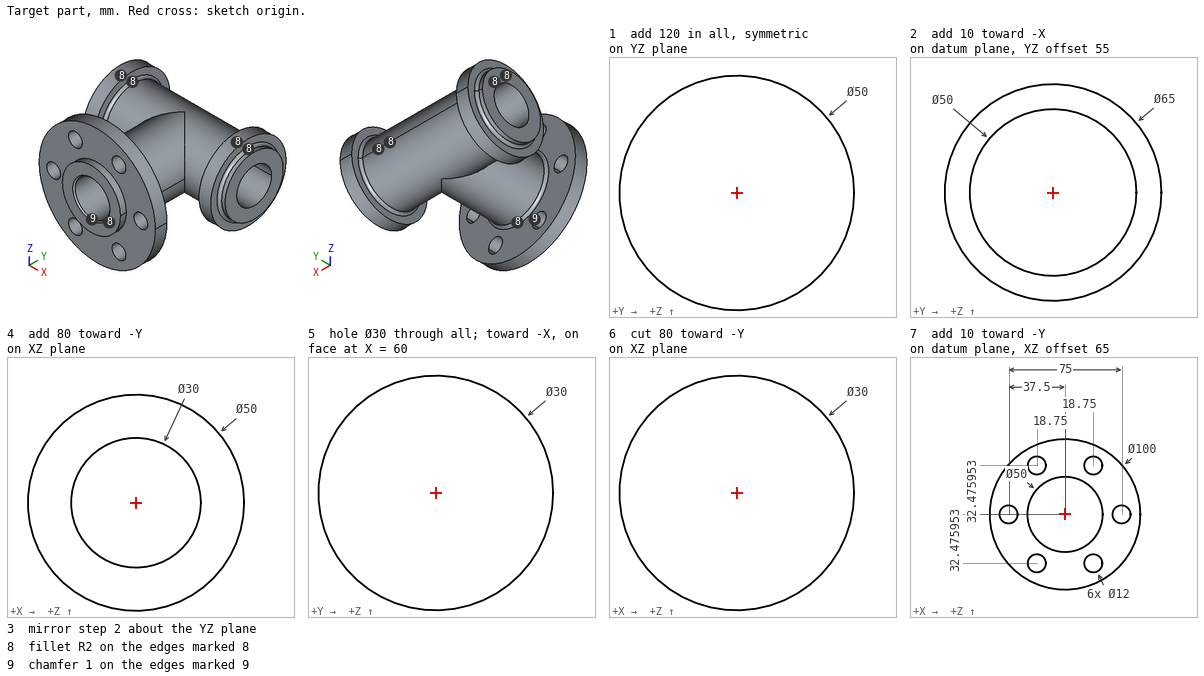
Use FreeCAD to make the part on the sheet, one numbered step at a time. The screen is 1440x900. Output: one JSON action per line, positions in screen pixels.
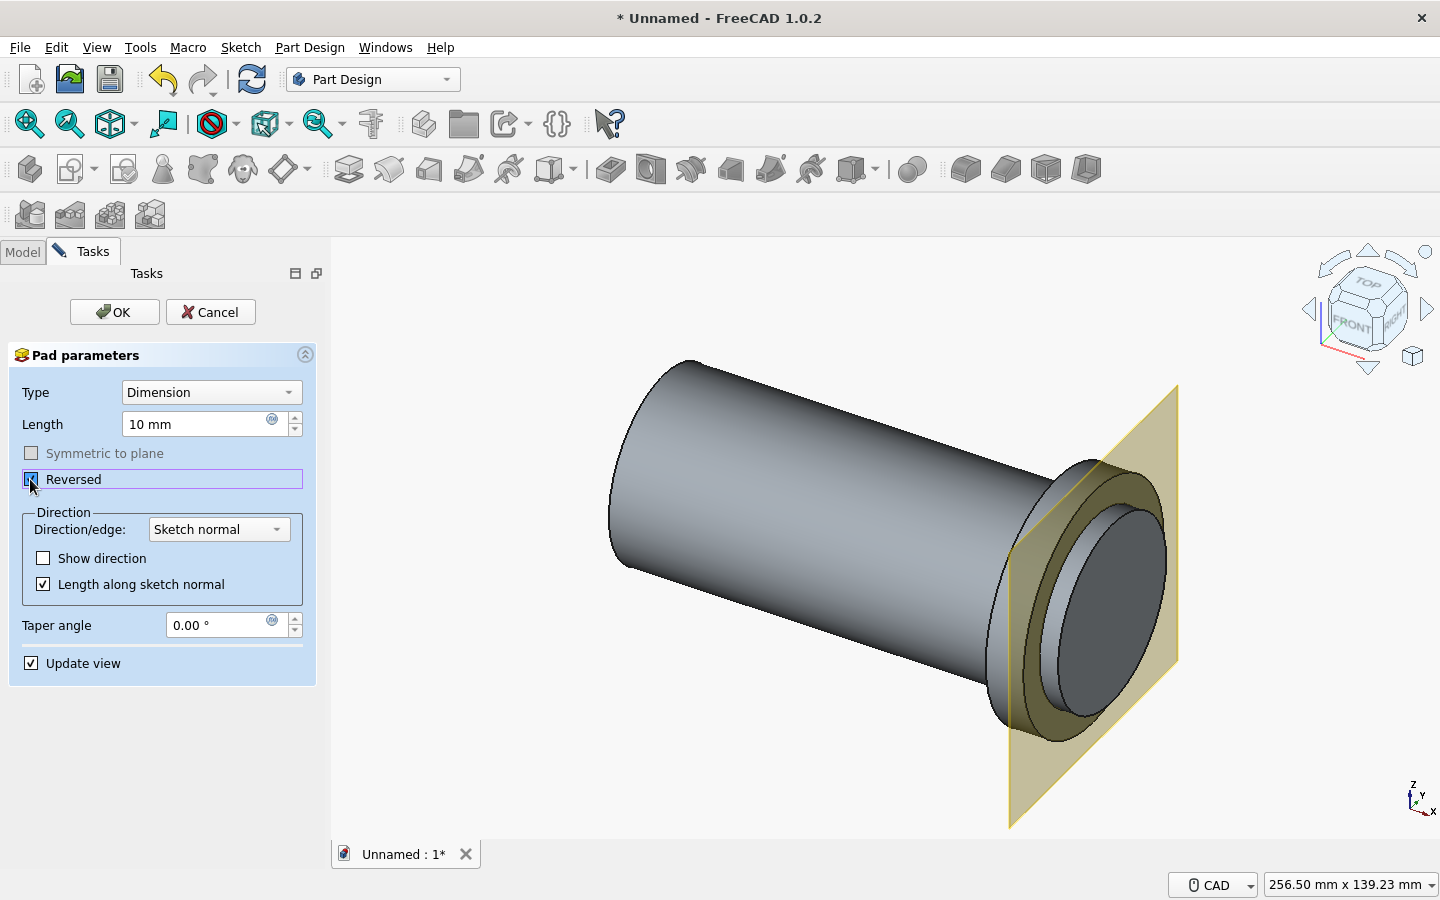
{"action": "left_click", "coordinate": [115, 312]}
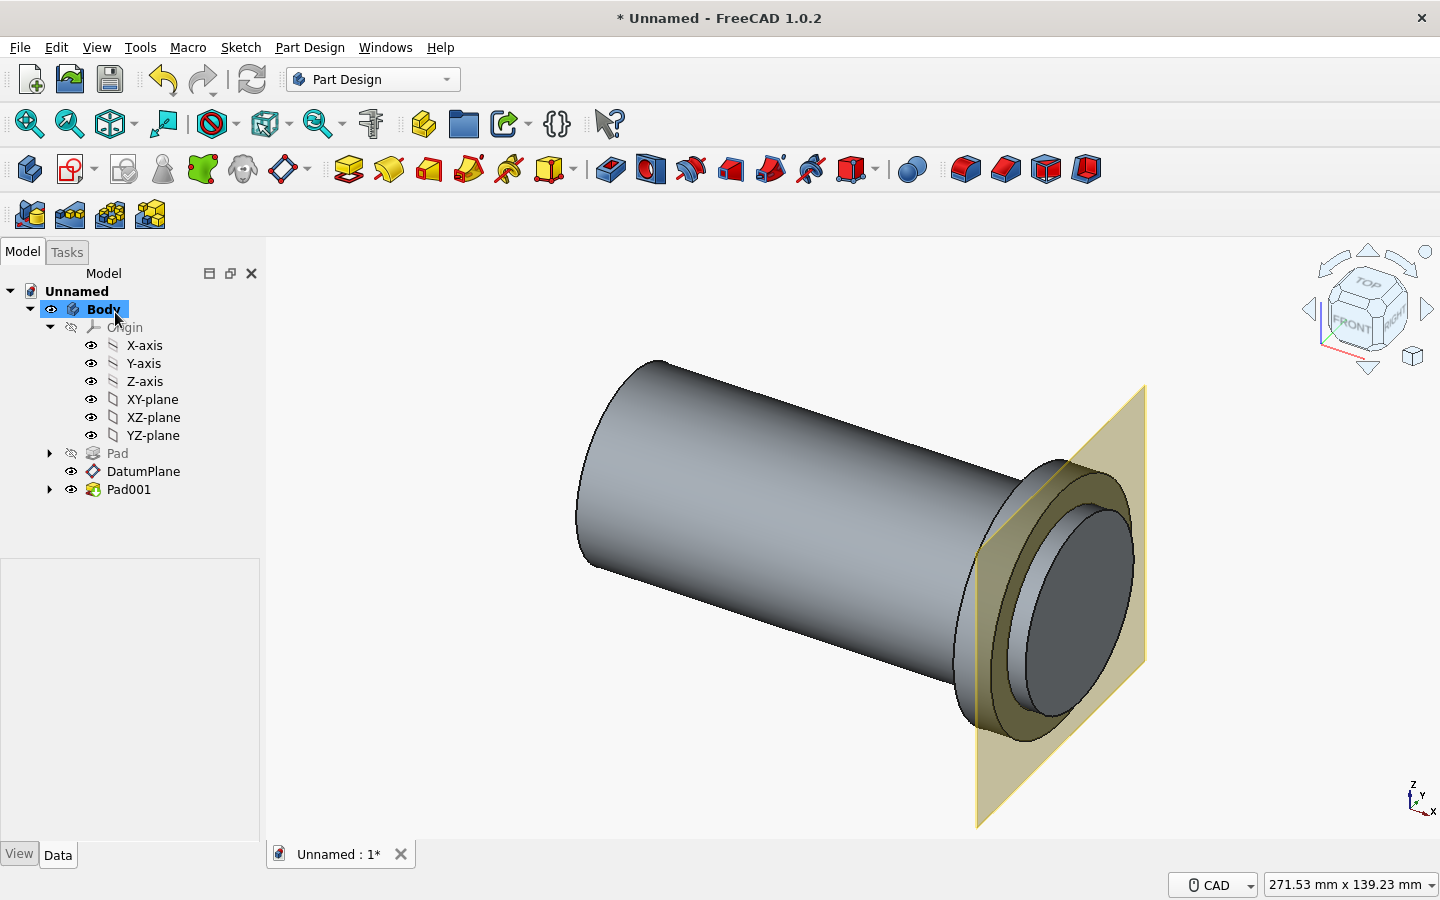
{"action": "left_click", "coordinate": [116, 471]}
{"action": "key", "text": "space"}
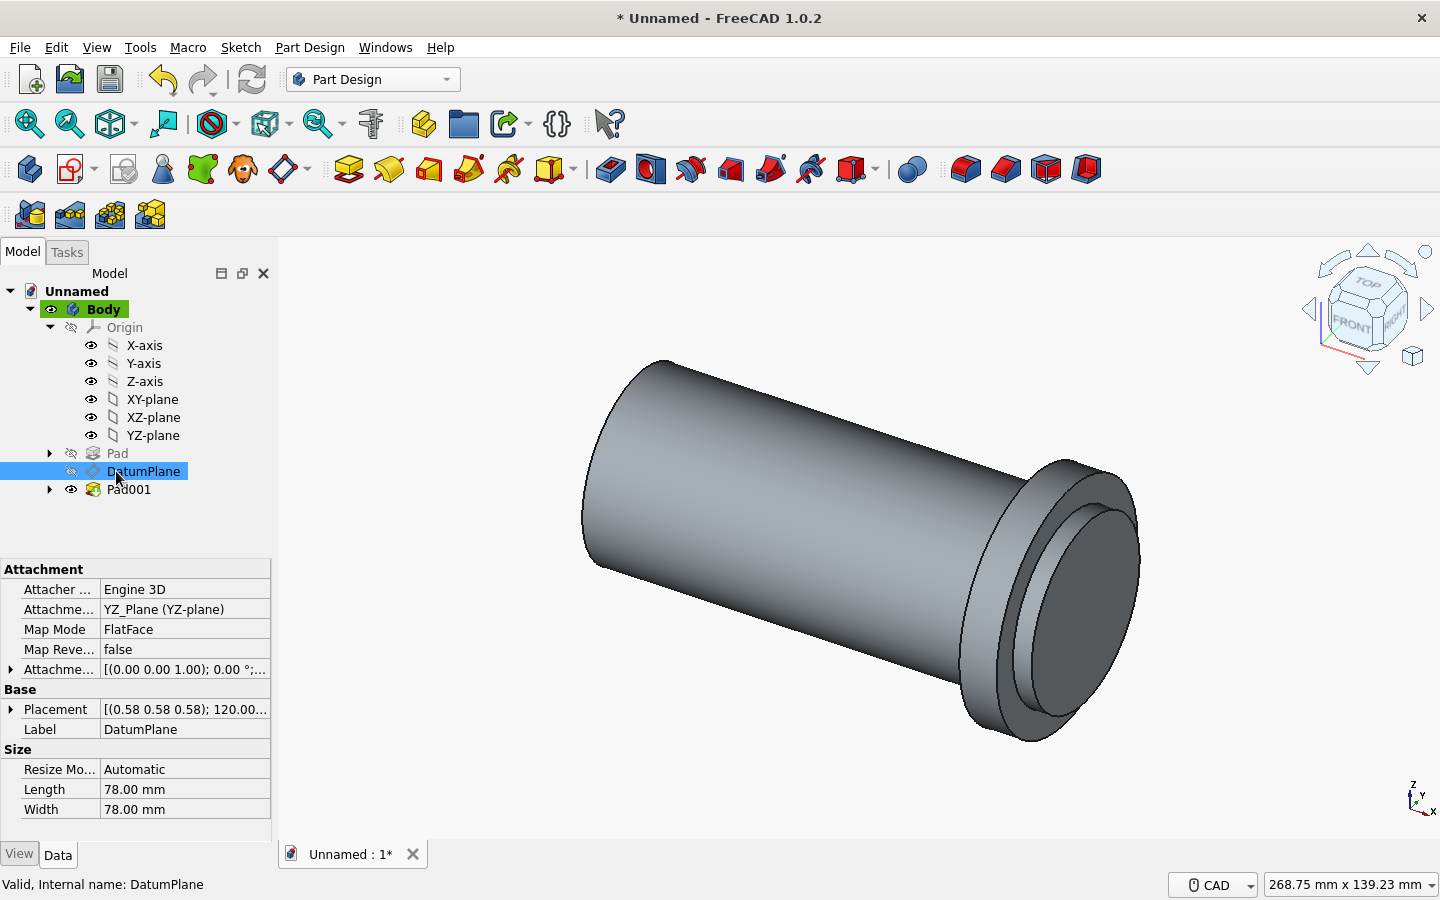
{"action": "left_click", "coordinate": [116, 489]}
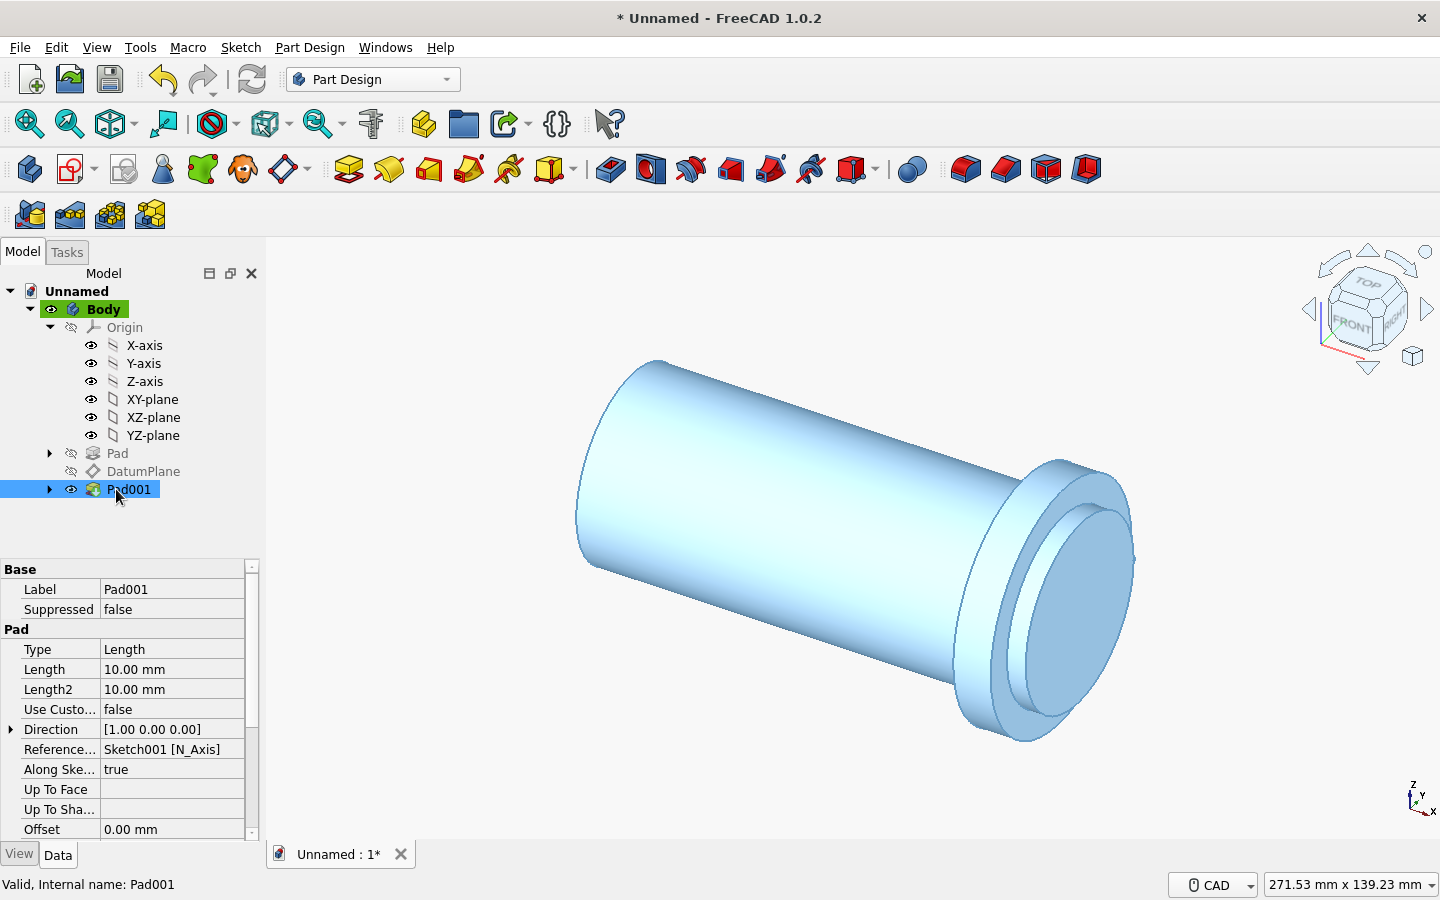
{"action": "left_click", "coordinate": [30, 214]}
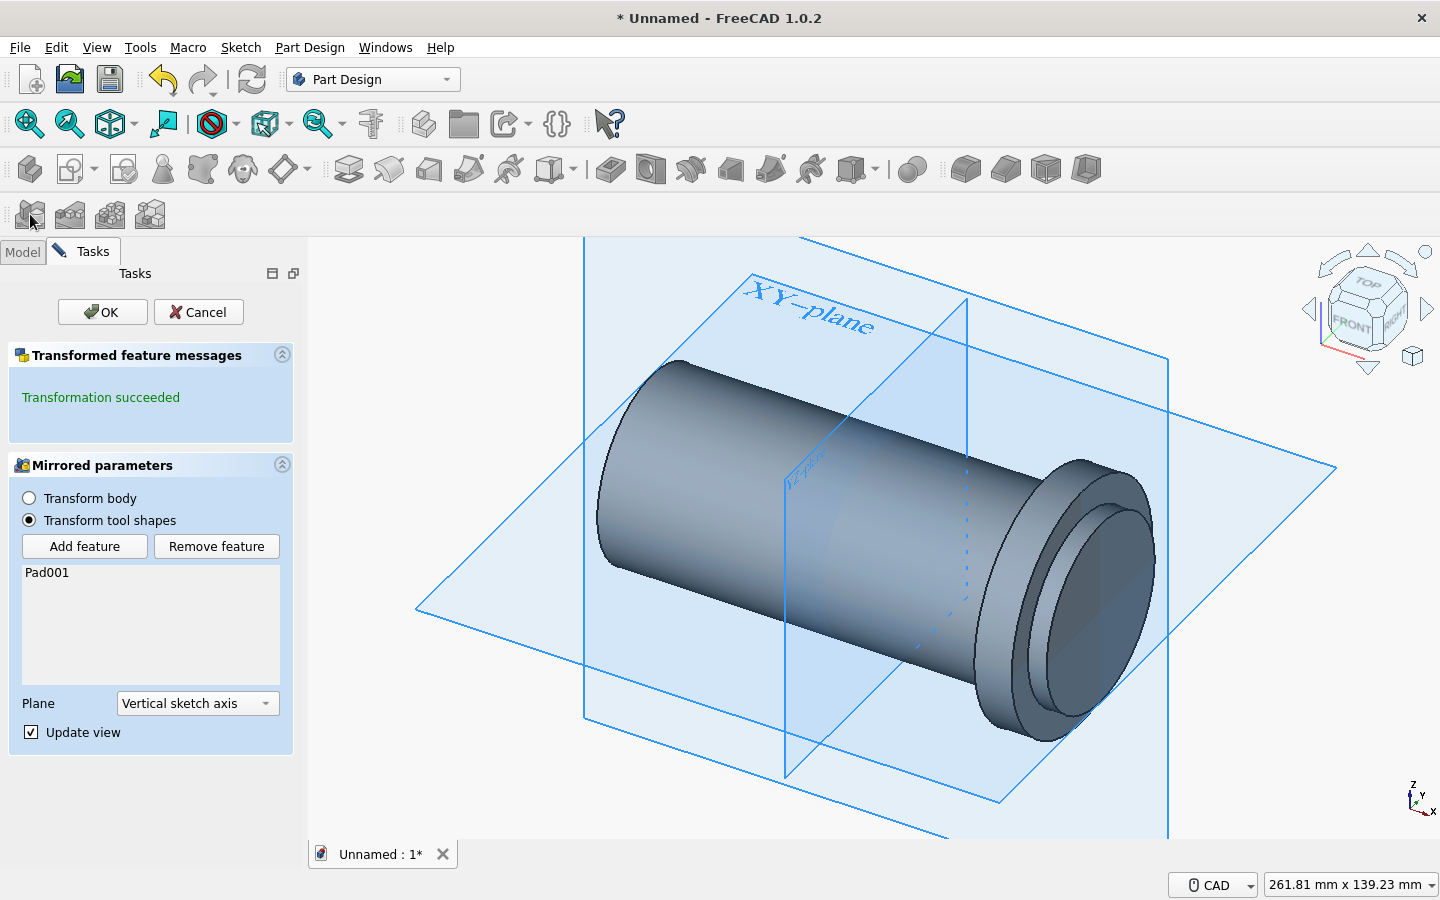
{"action": "left_click", "coordinate": [198, 704]}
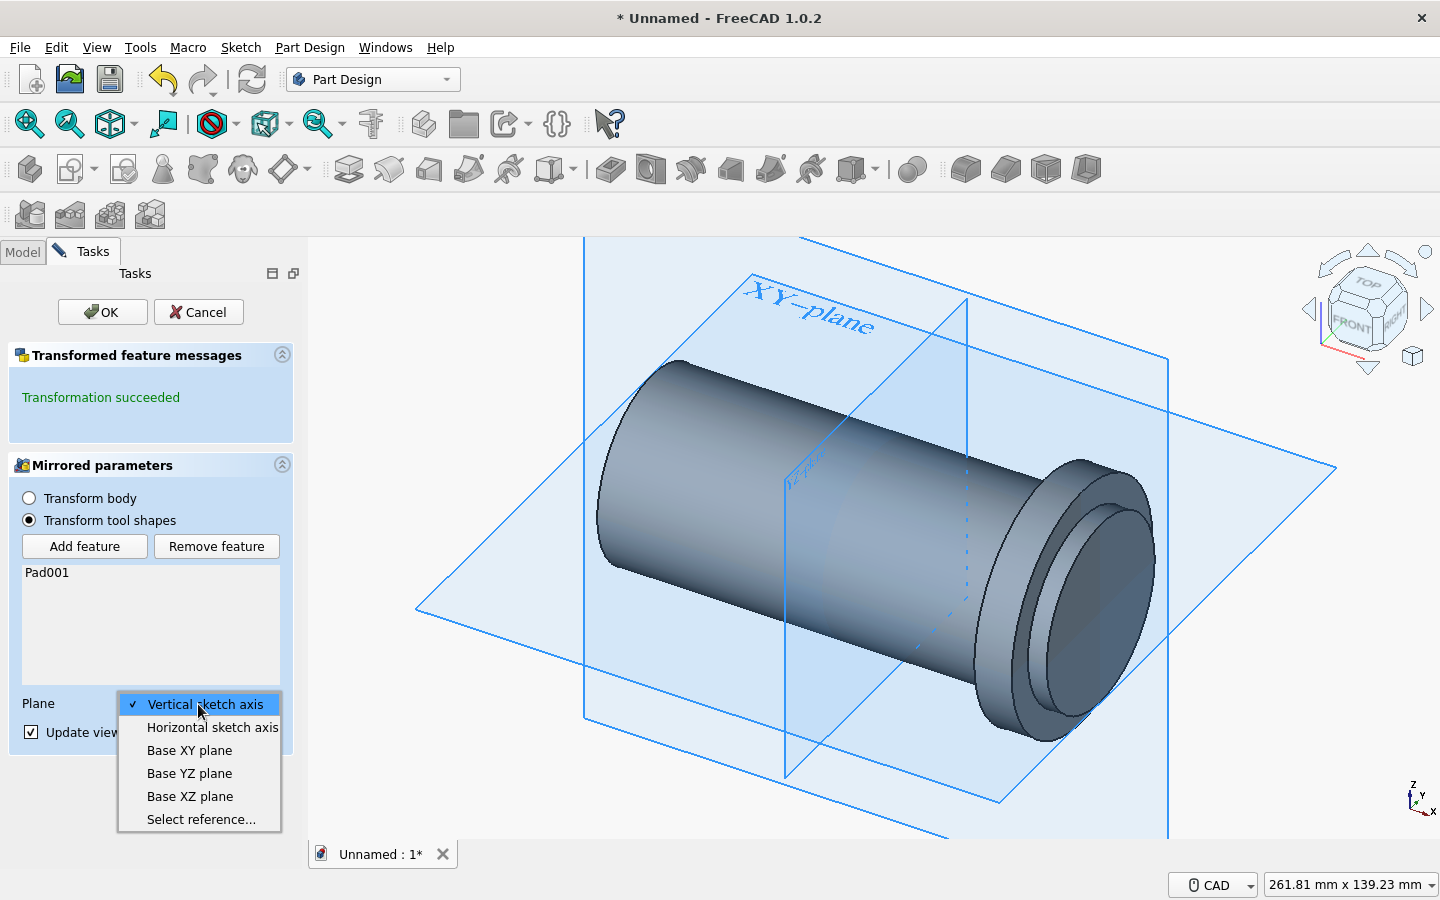
{"action": "left_click", "coordinate": [198, 774]}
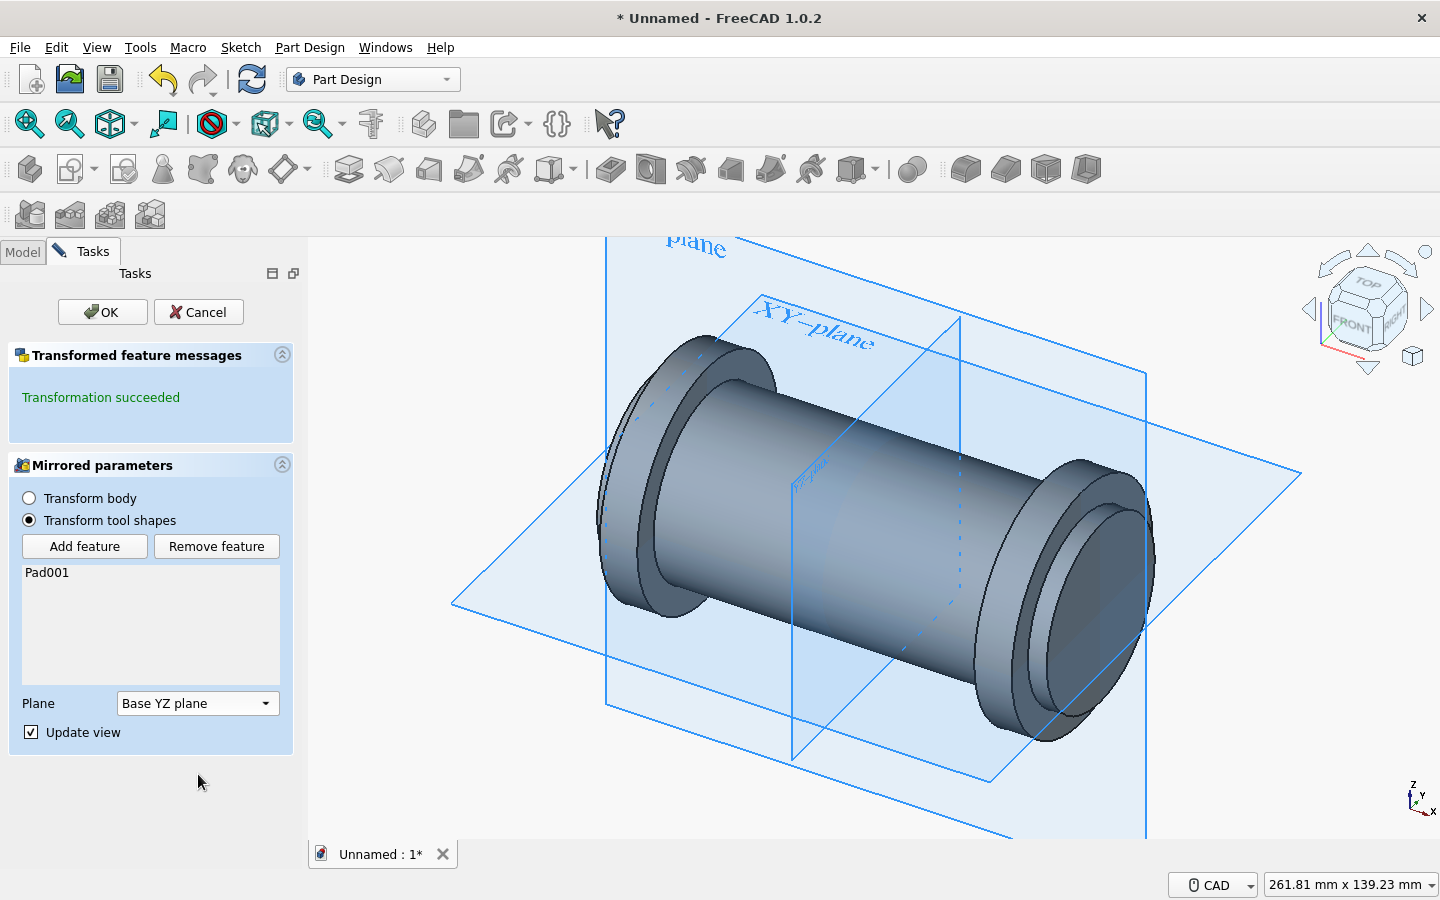
{"action": "left_click", "coordinate": [103, 312]}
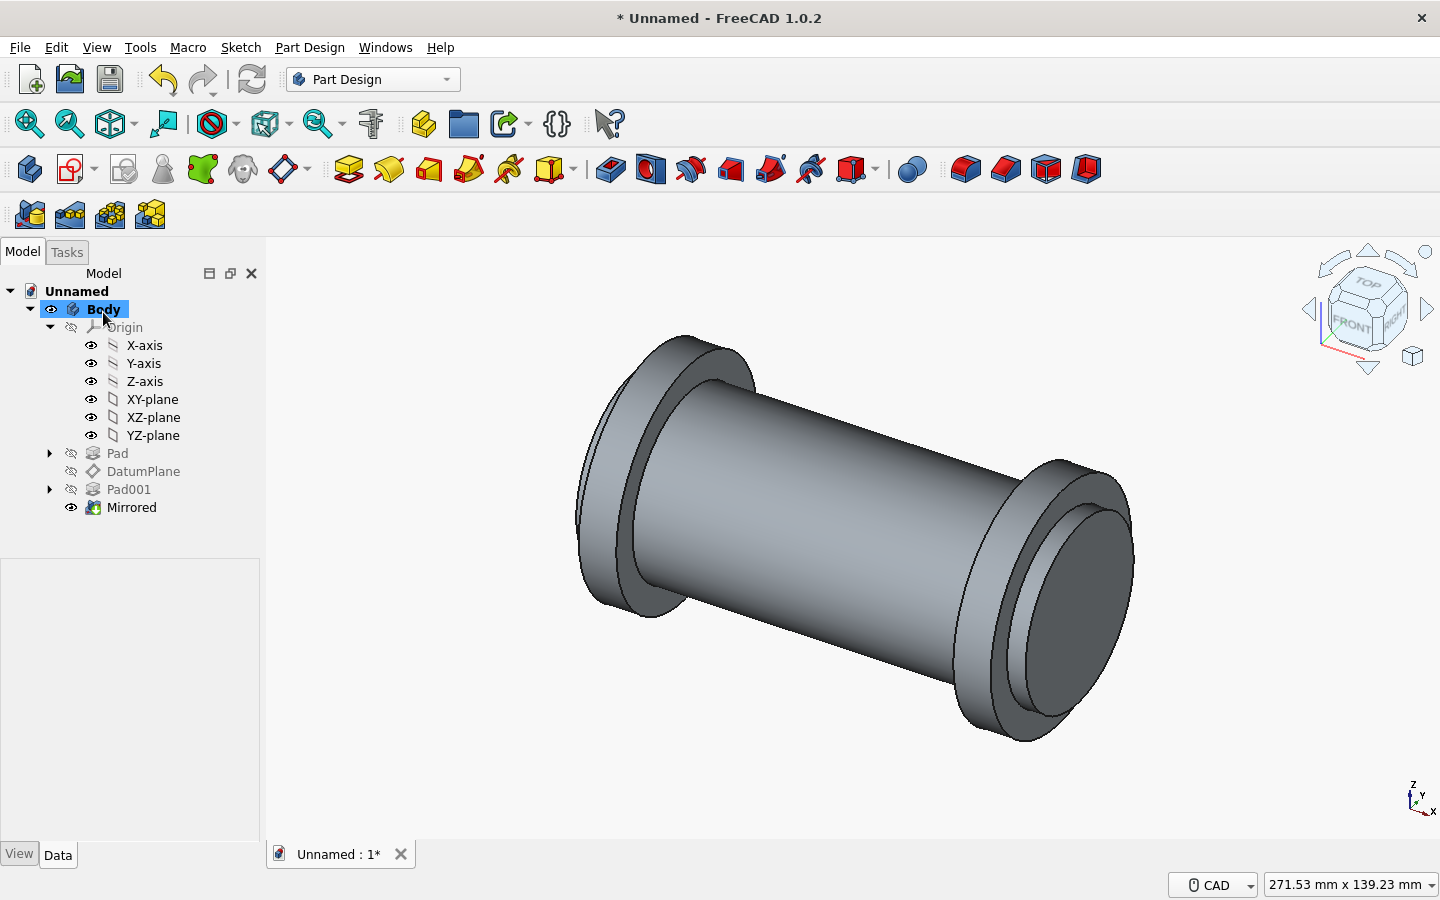
{"action": "left_click", "coordinate": [70, 170]}